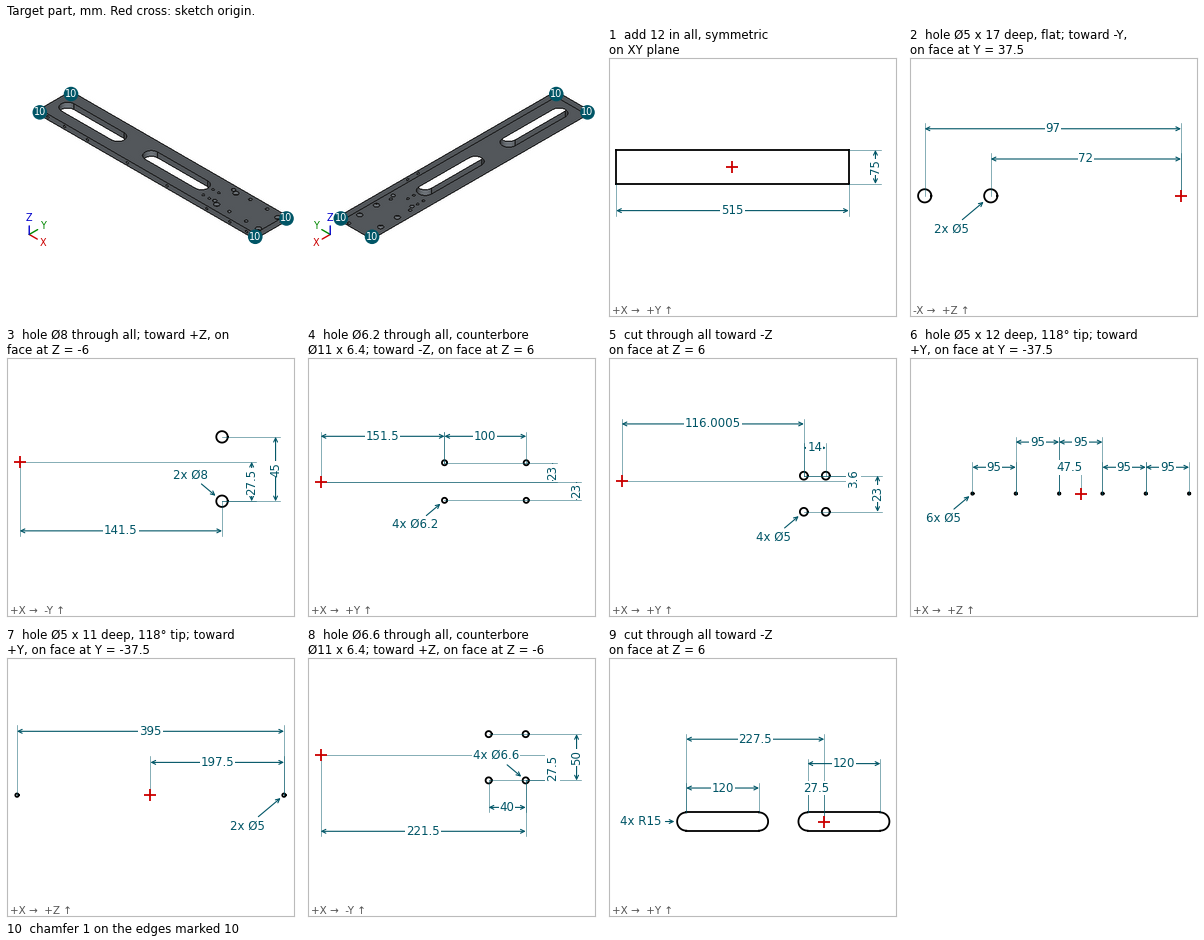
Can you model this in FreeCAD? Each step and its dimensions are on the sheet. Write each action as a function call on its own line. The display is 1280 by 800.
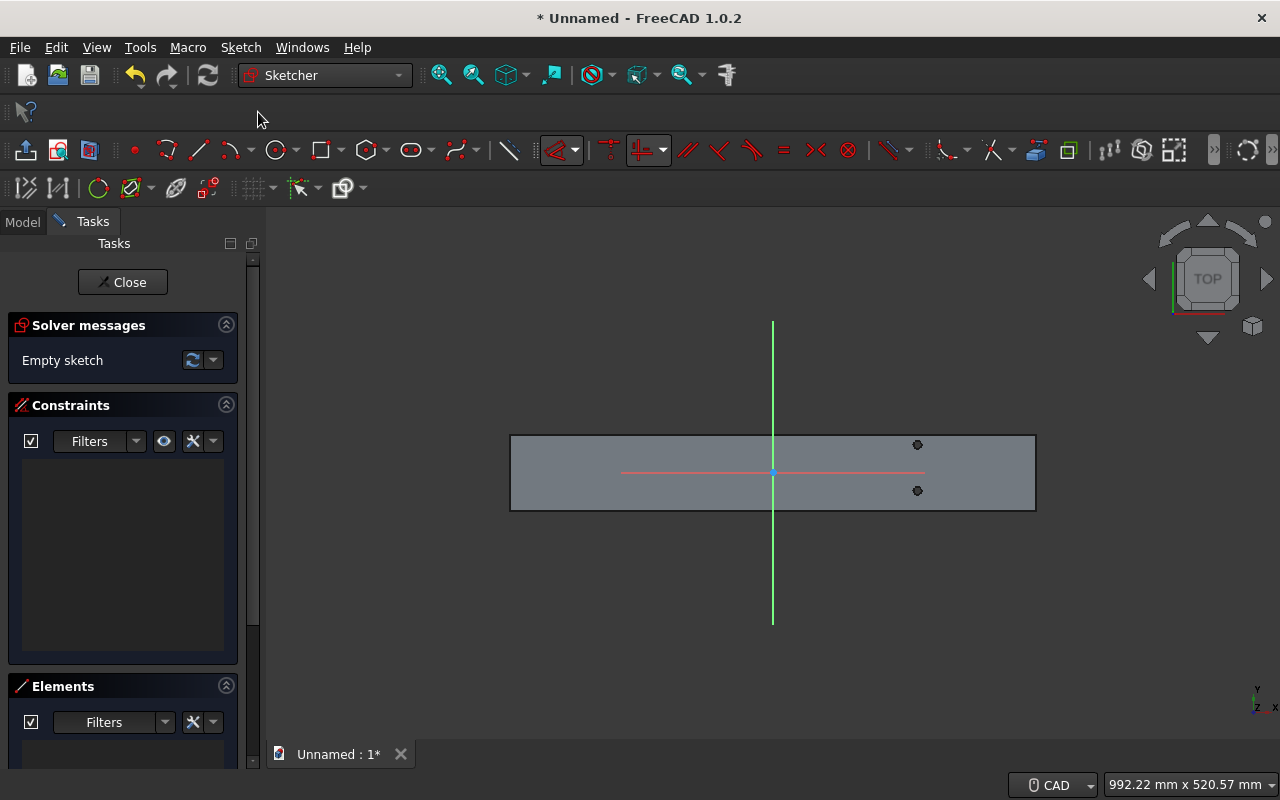
scroll(1065, 473, up, 4)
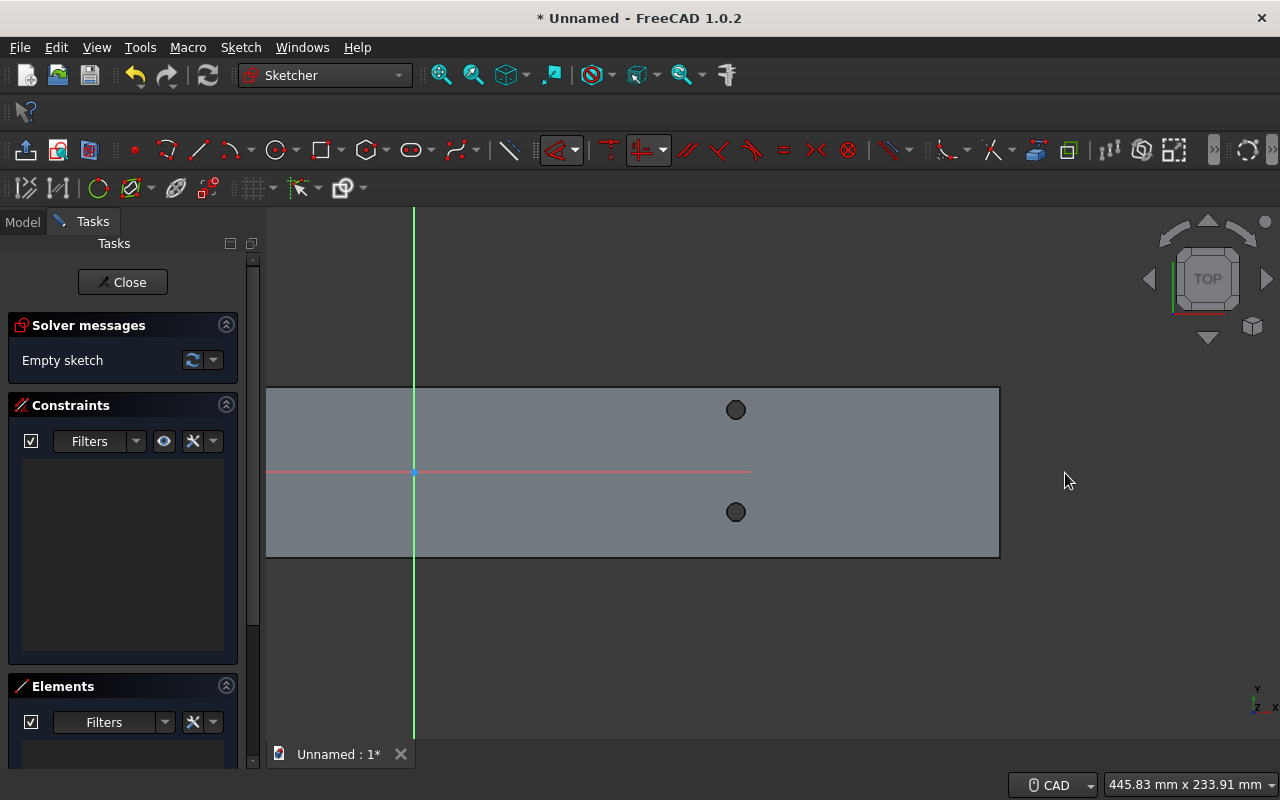
click(276, 150)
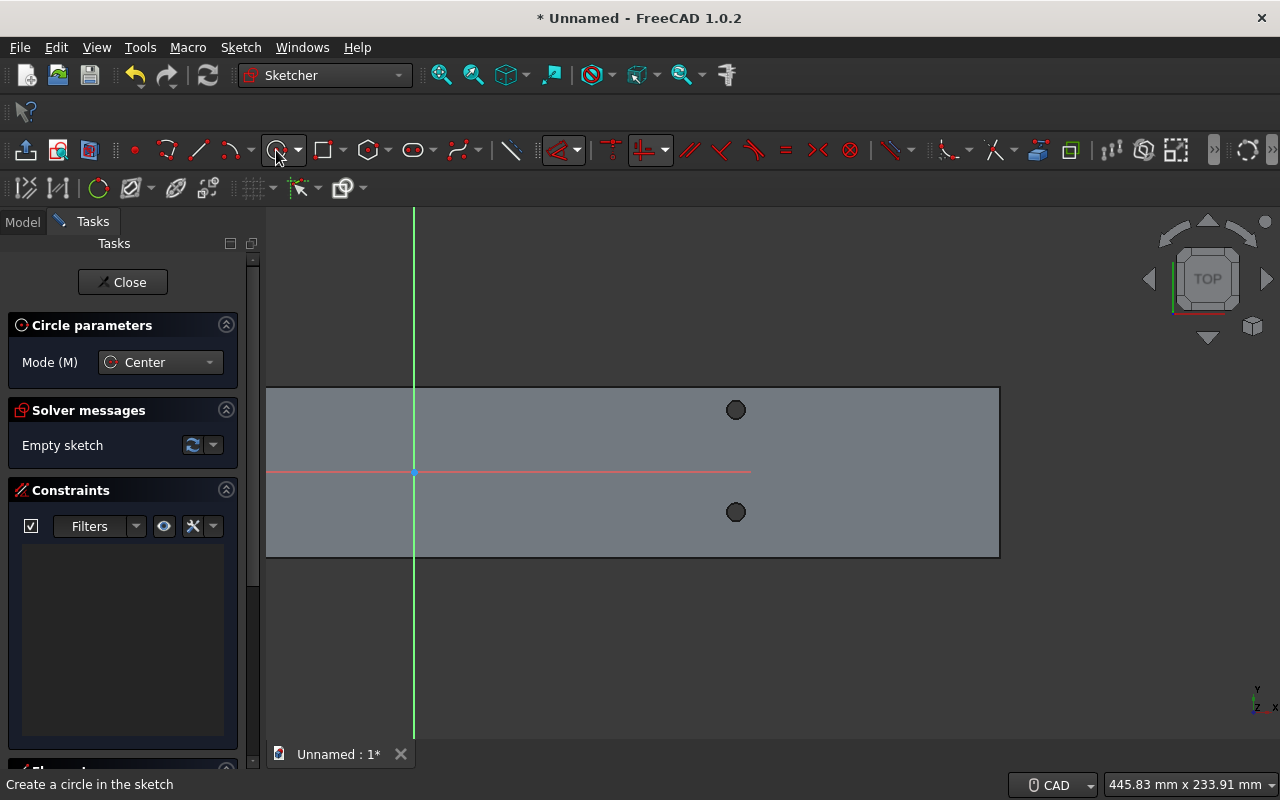
scroll(759, 420, up, 6)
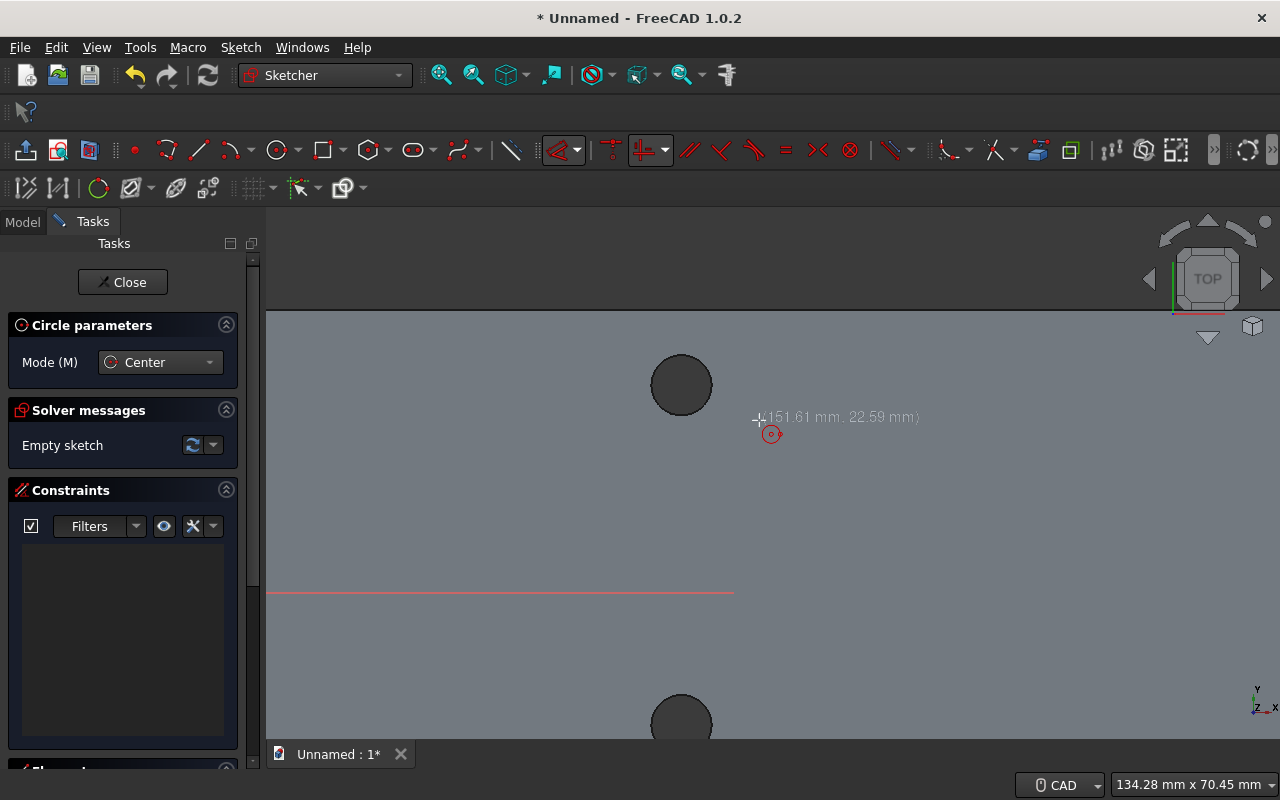
click(757, 419)
click(774, 403)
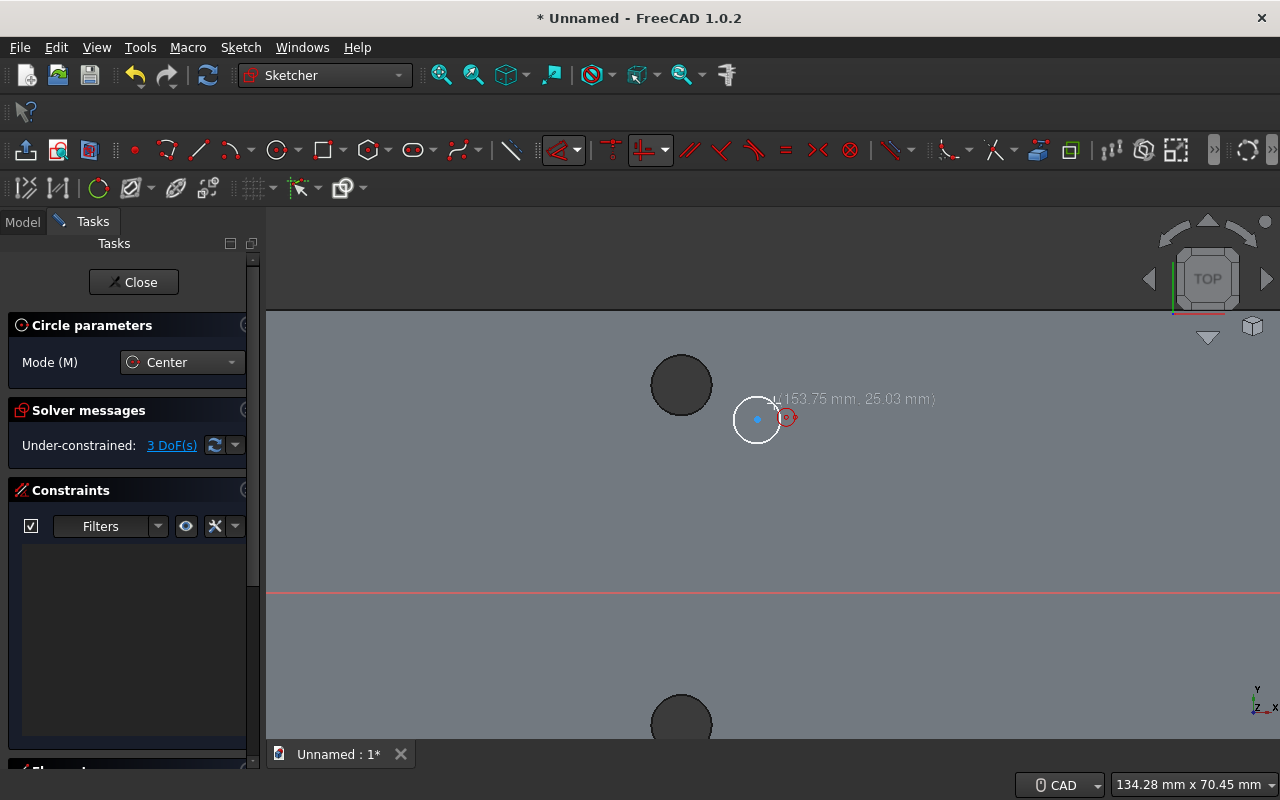
scroll(761, 421, down, 6)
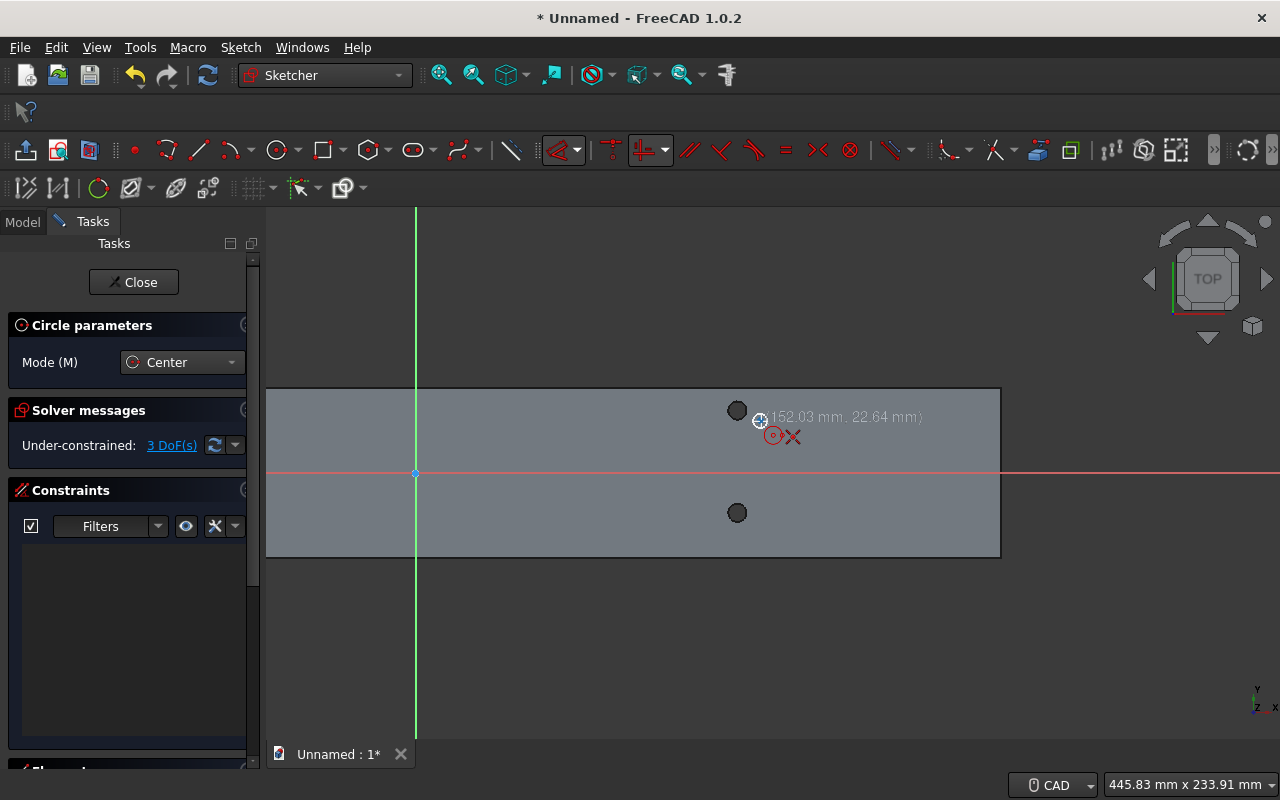
scroll(760, 525, up, 6)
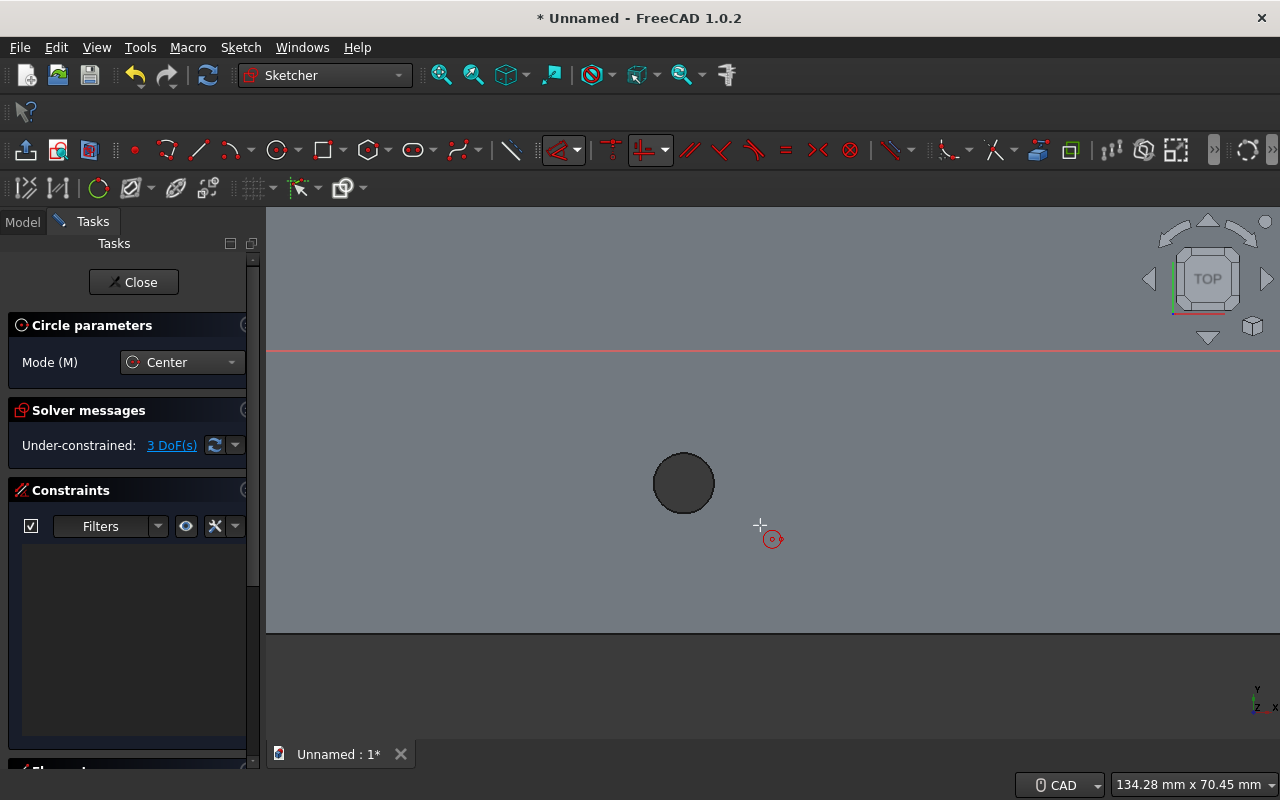
click(759, 525)
click(776, 508)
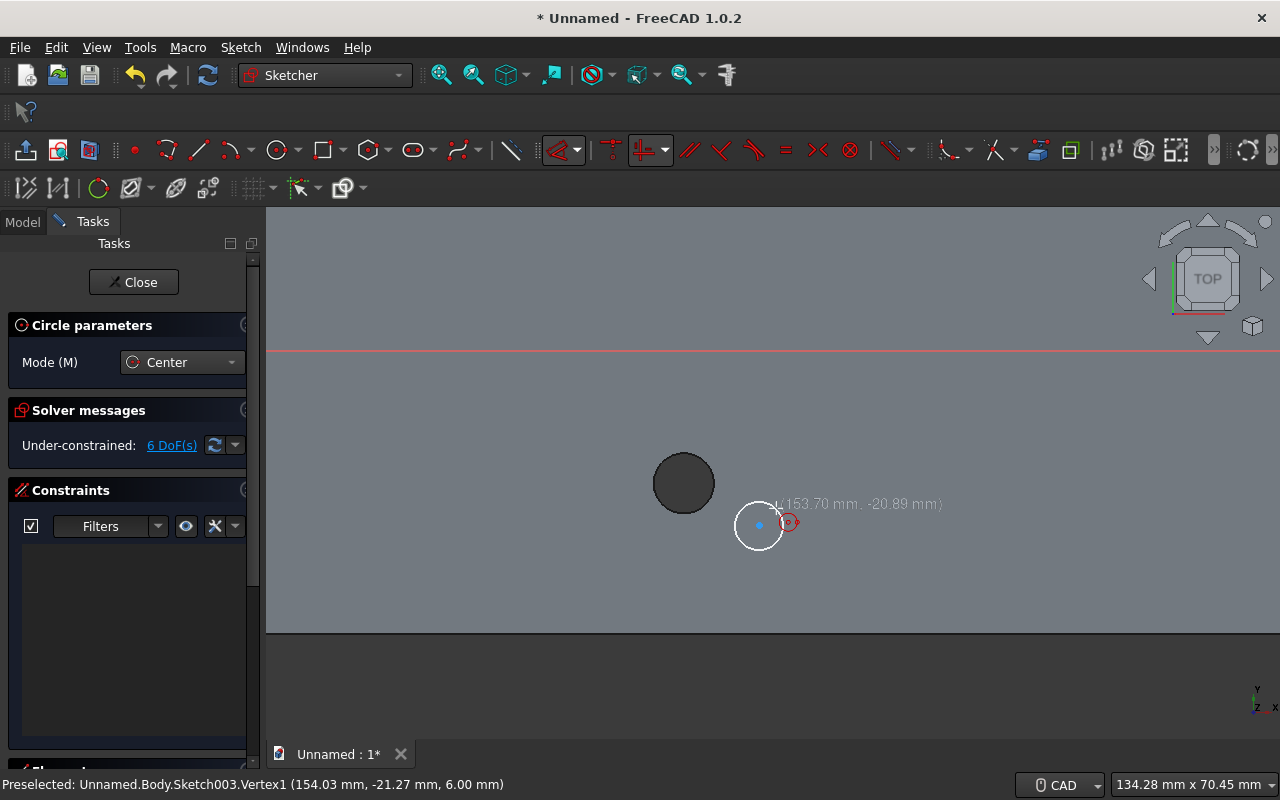
scroll(760, 525, down, 6)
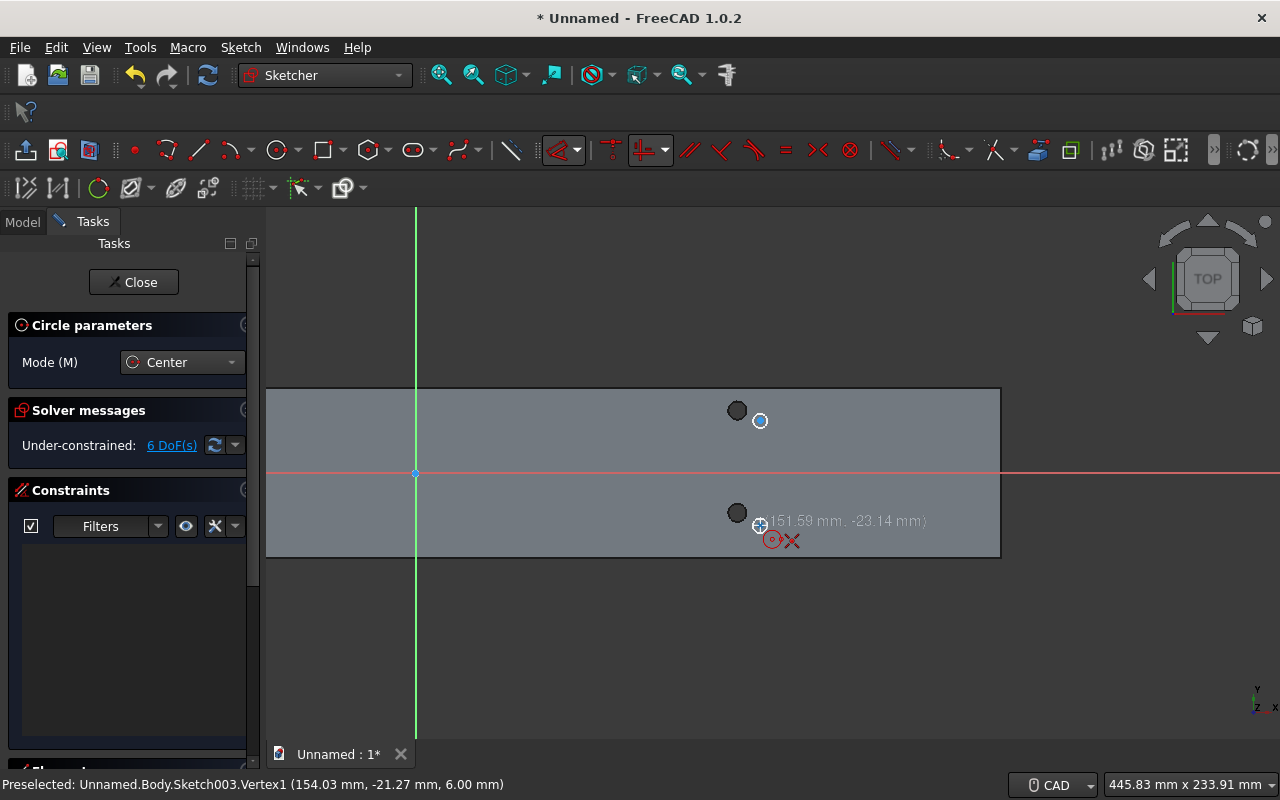
scroll(988, 421, up, 6)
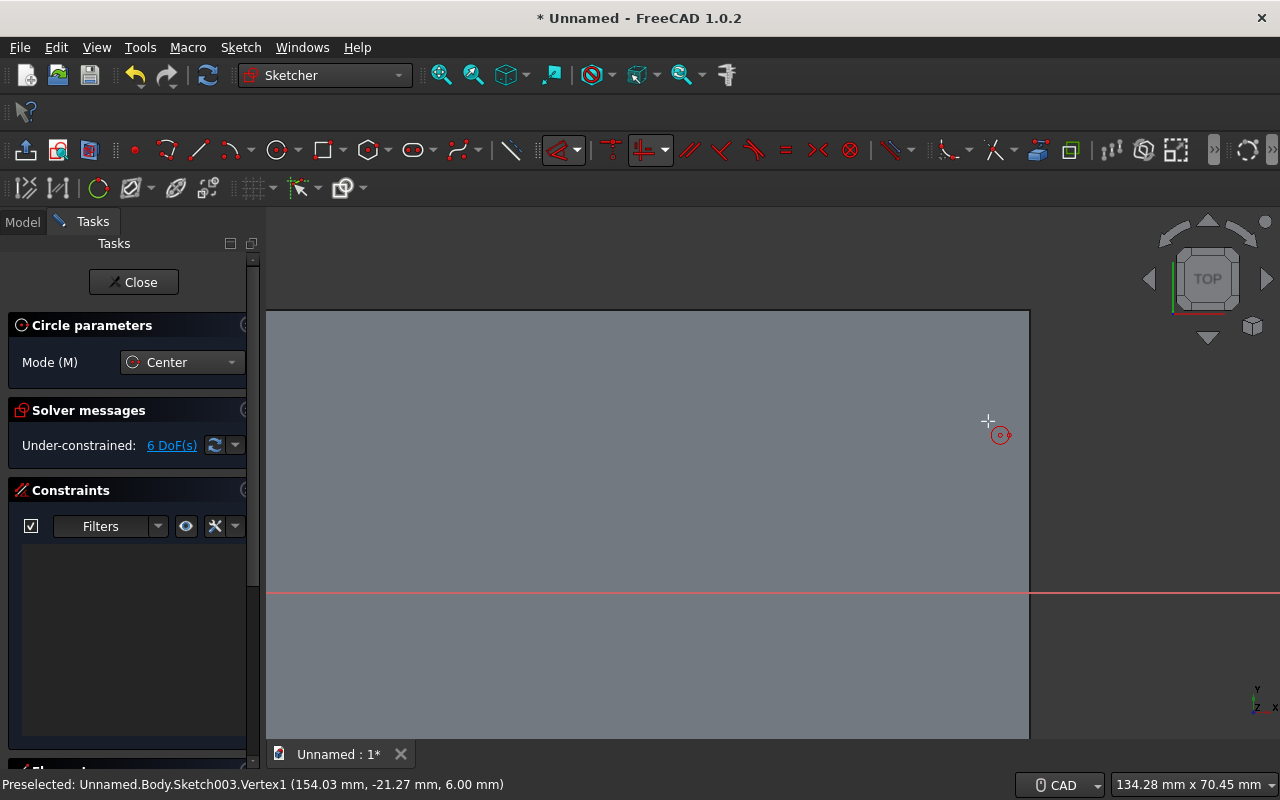
click(985, 419)
click(1002, 403)